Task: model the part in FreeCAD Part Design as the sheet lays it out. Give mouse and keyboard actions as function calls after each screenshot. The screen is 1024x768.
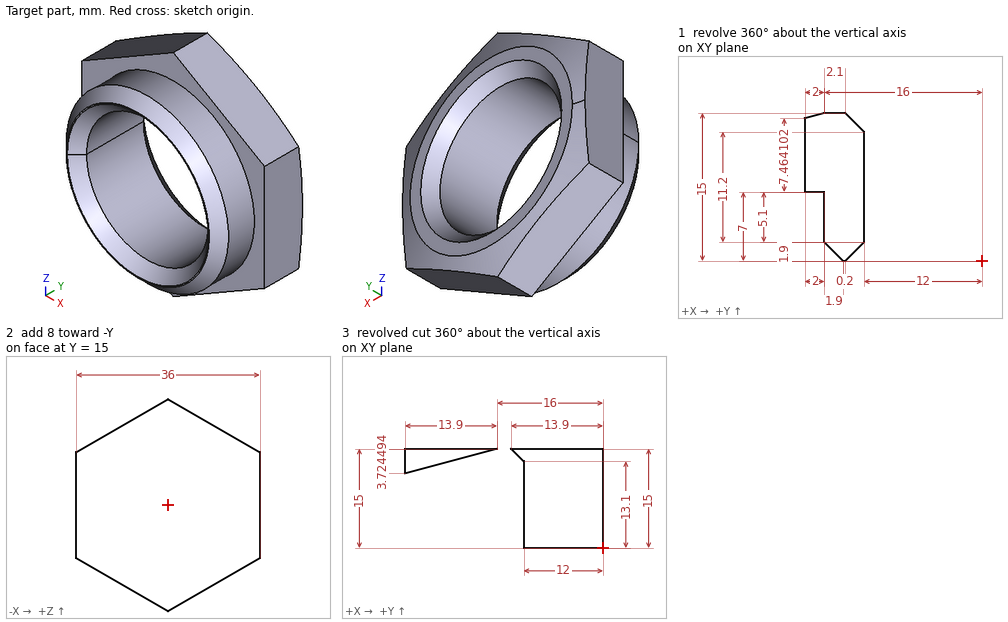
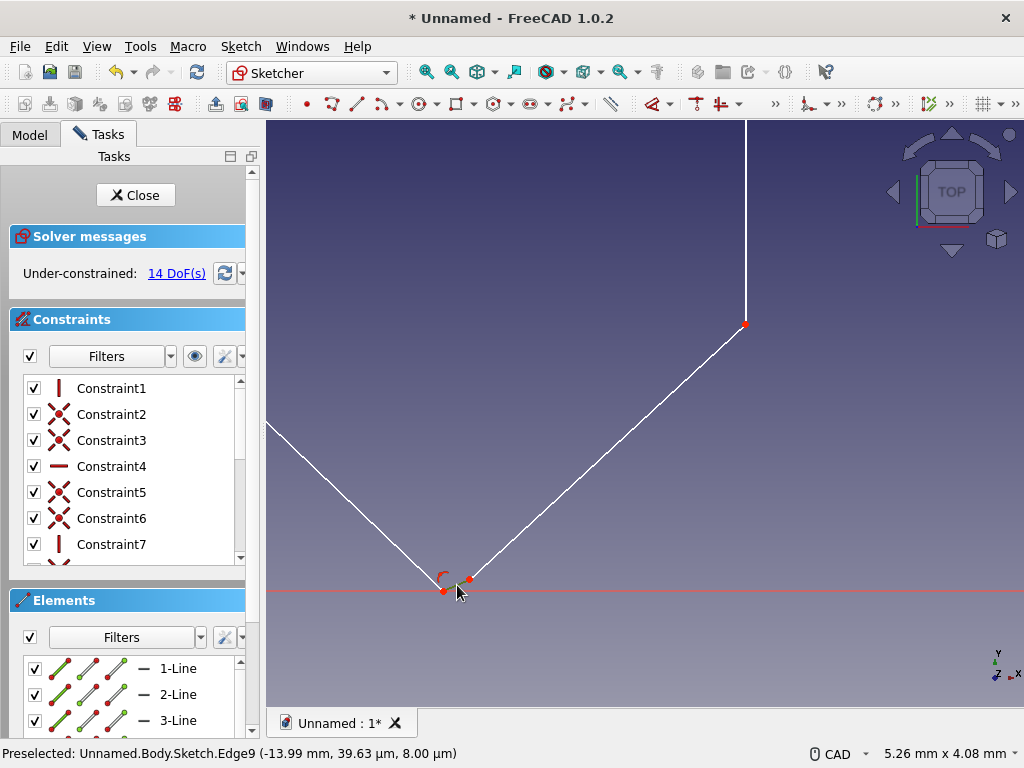
key(h)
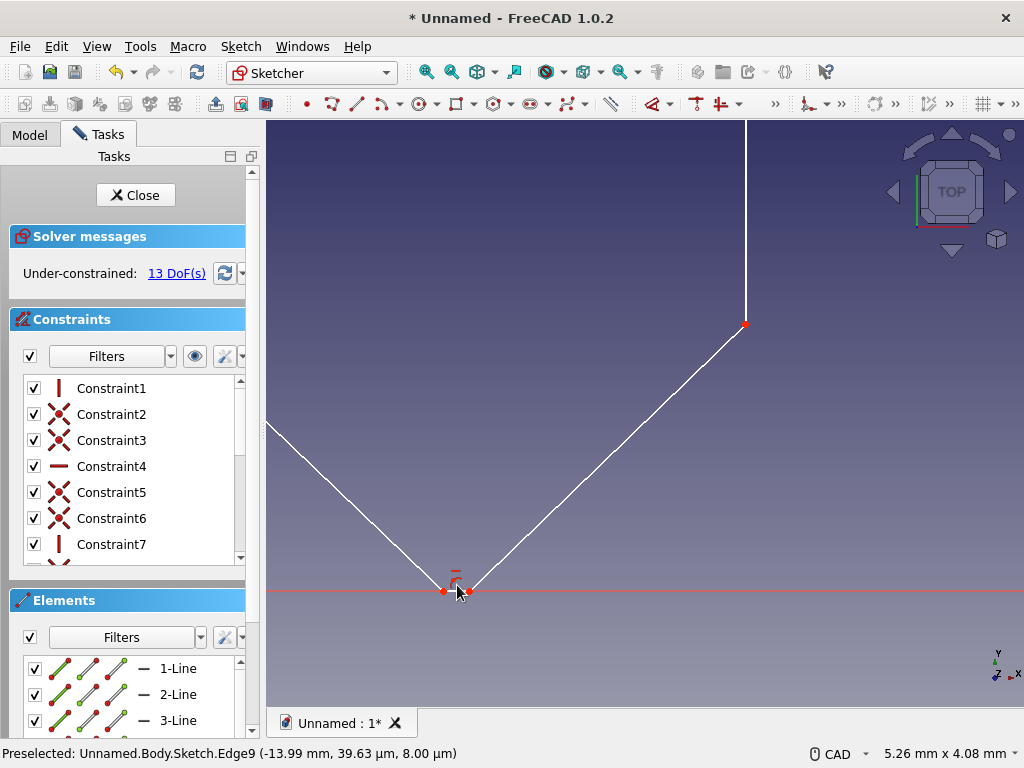
click(652, 104)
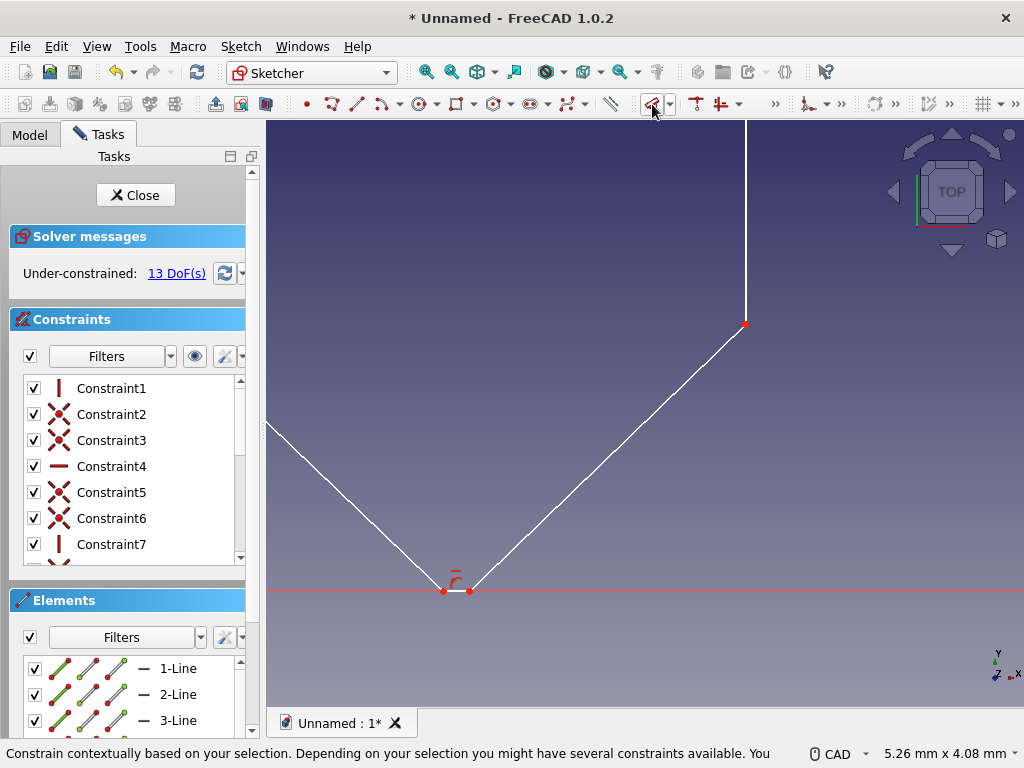
scroll(458, 592, down, 9)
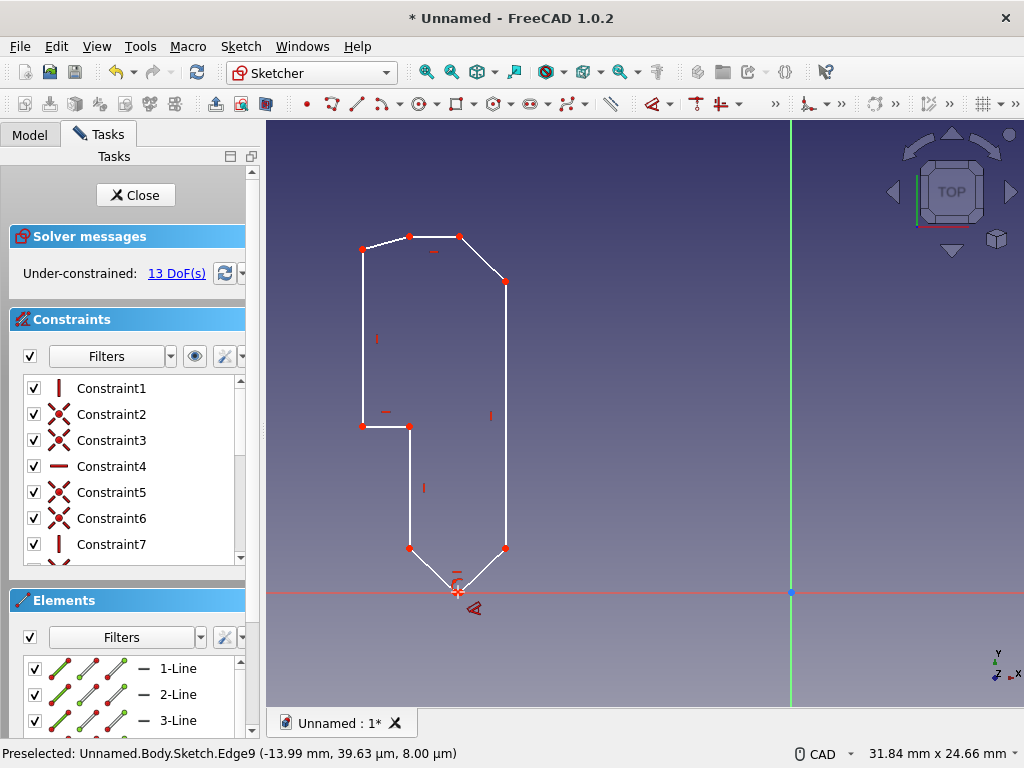
click(377, 427)
click(386, 461)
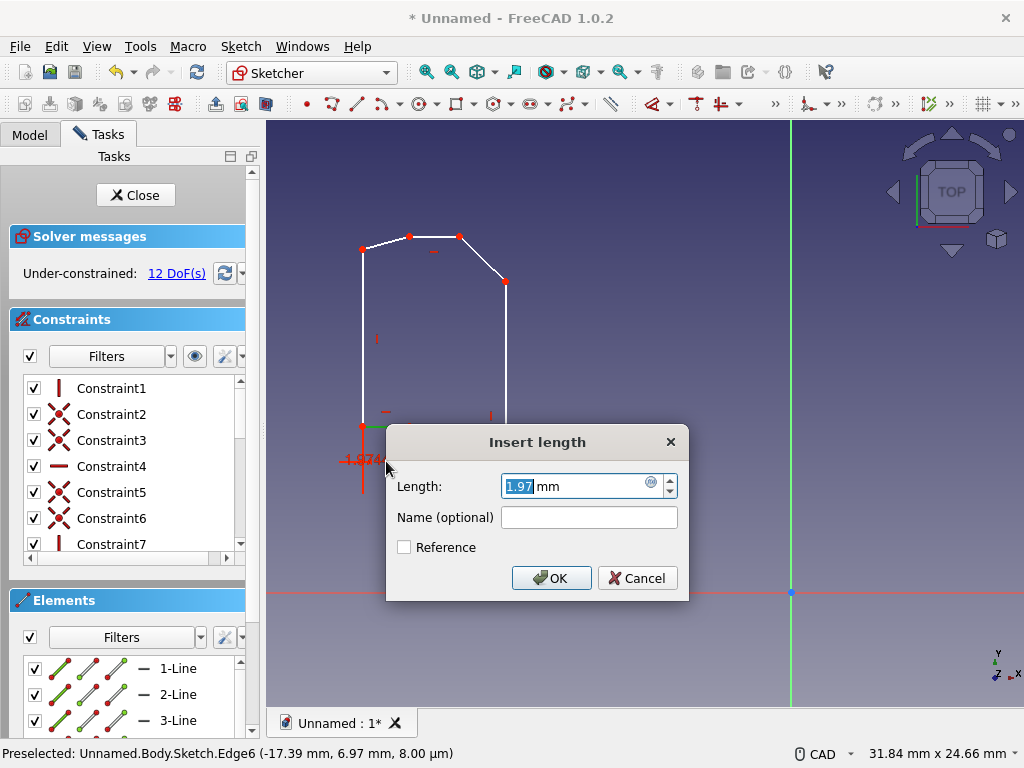
text(2)
key(Return)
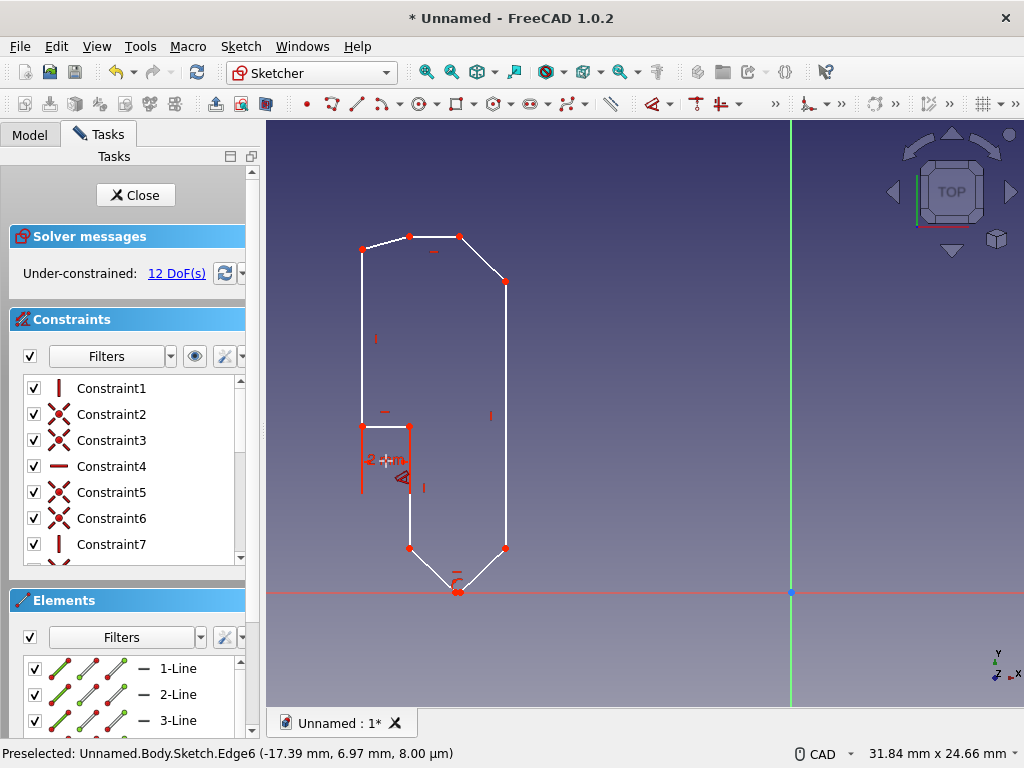
click(362, 427)
click(328, 510)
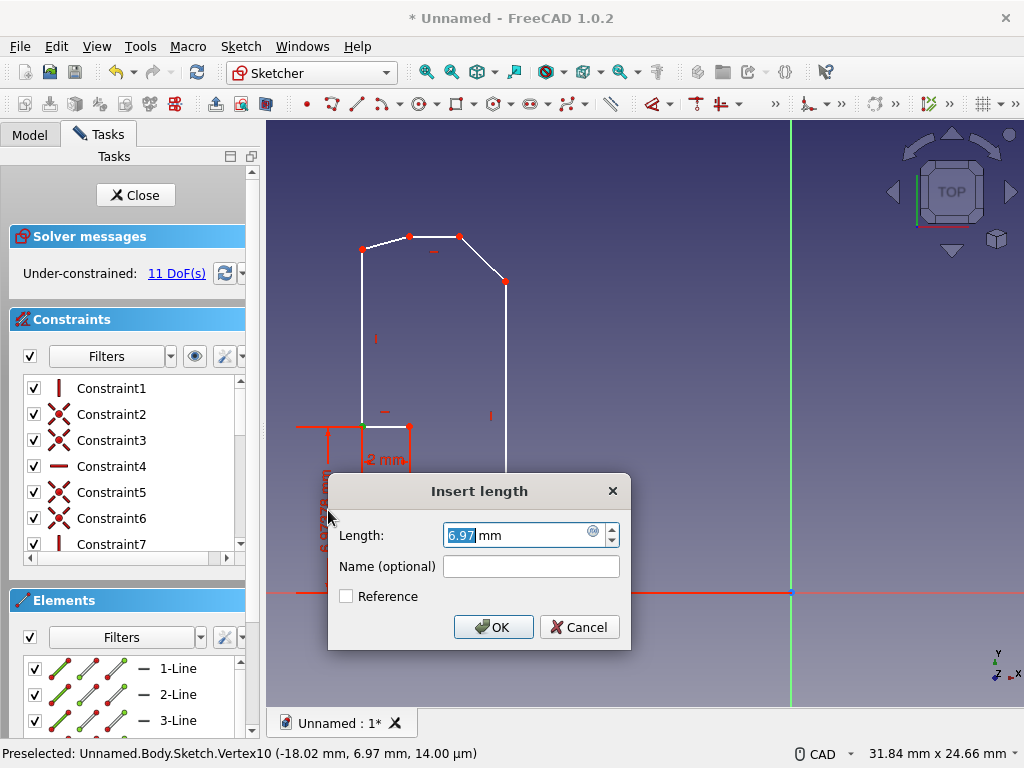
text(7)
key(Return)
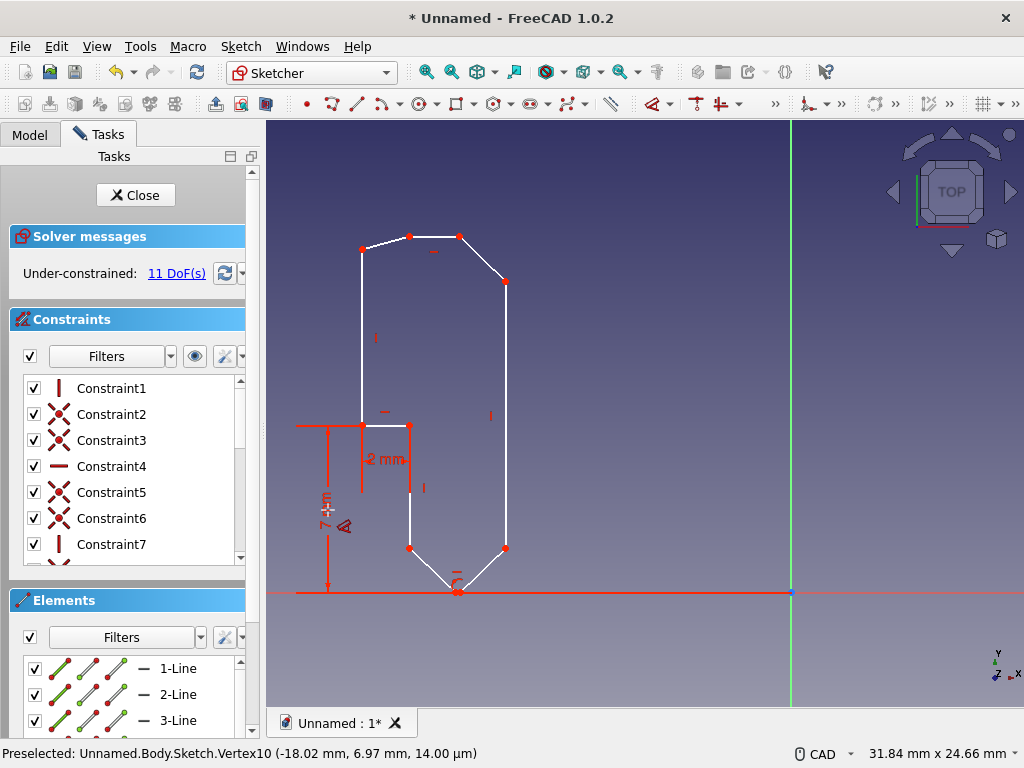
click(395, 240)
click(386, 203)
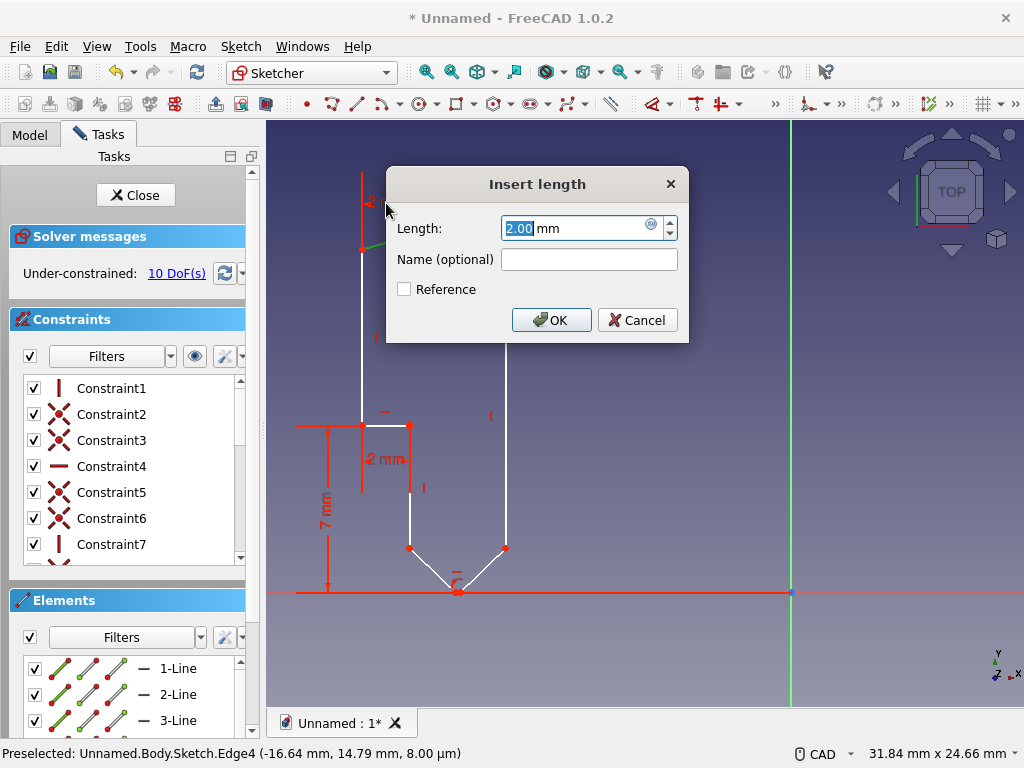
text(2)
key(Return)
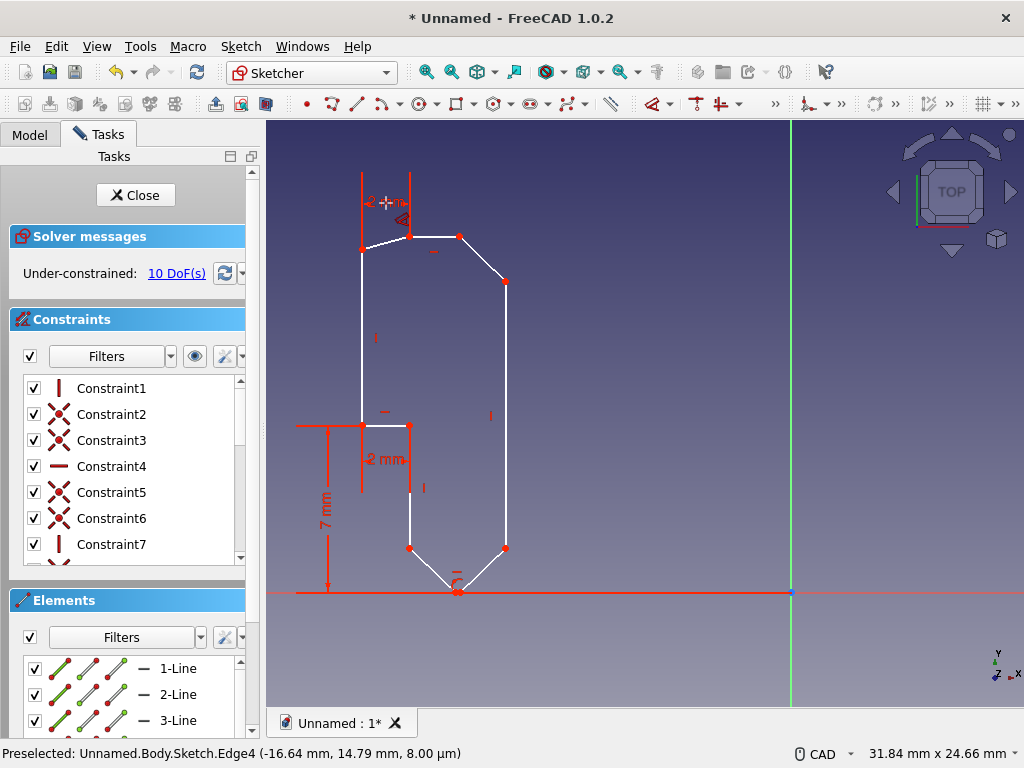
click(445, 237)
click(435, 271)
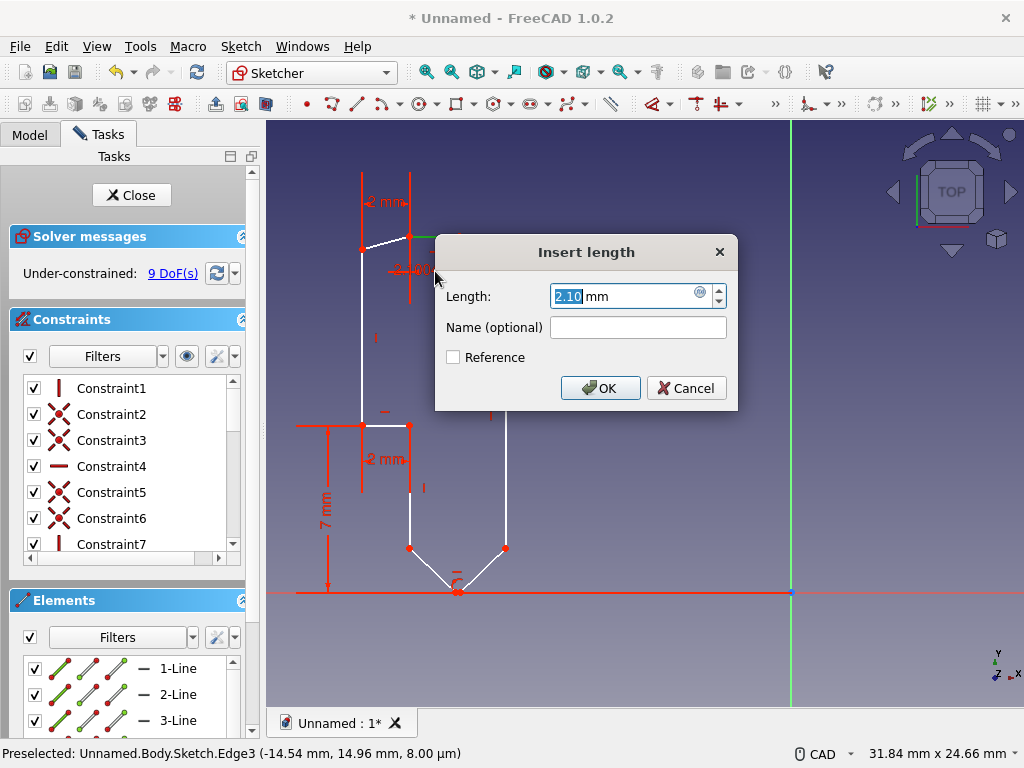
text(2.1)
key(Return)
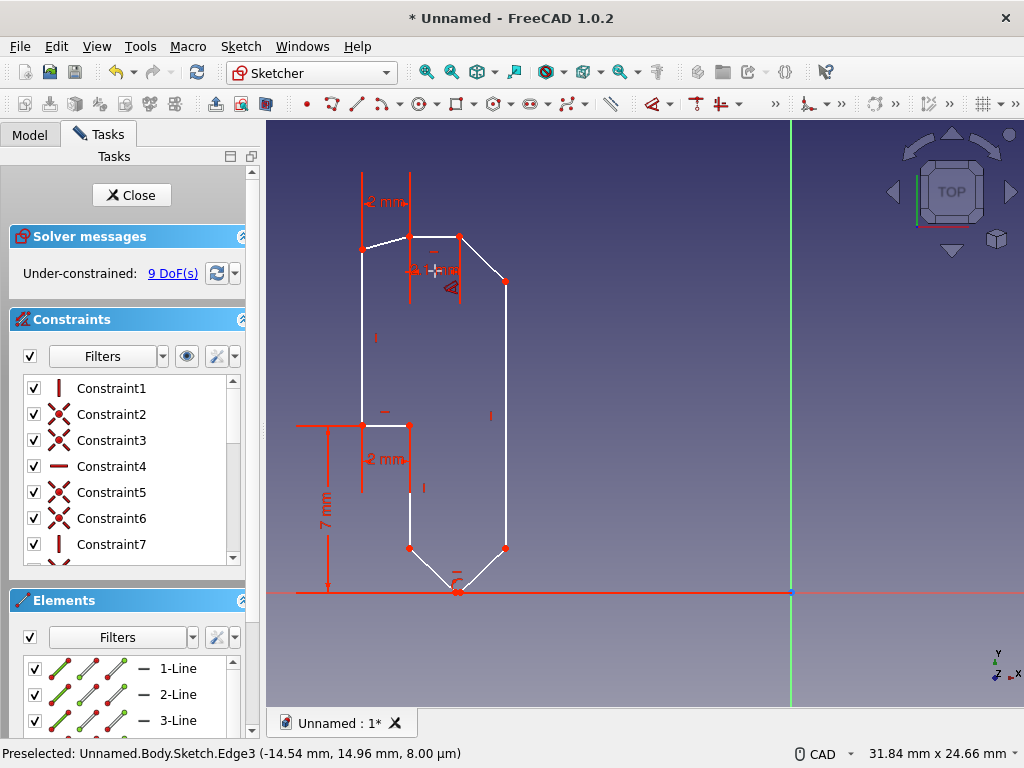
click(410, 463)
click(376, 487)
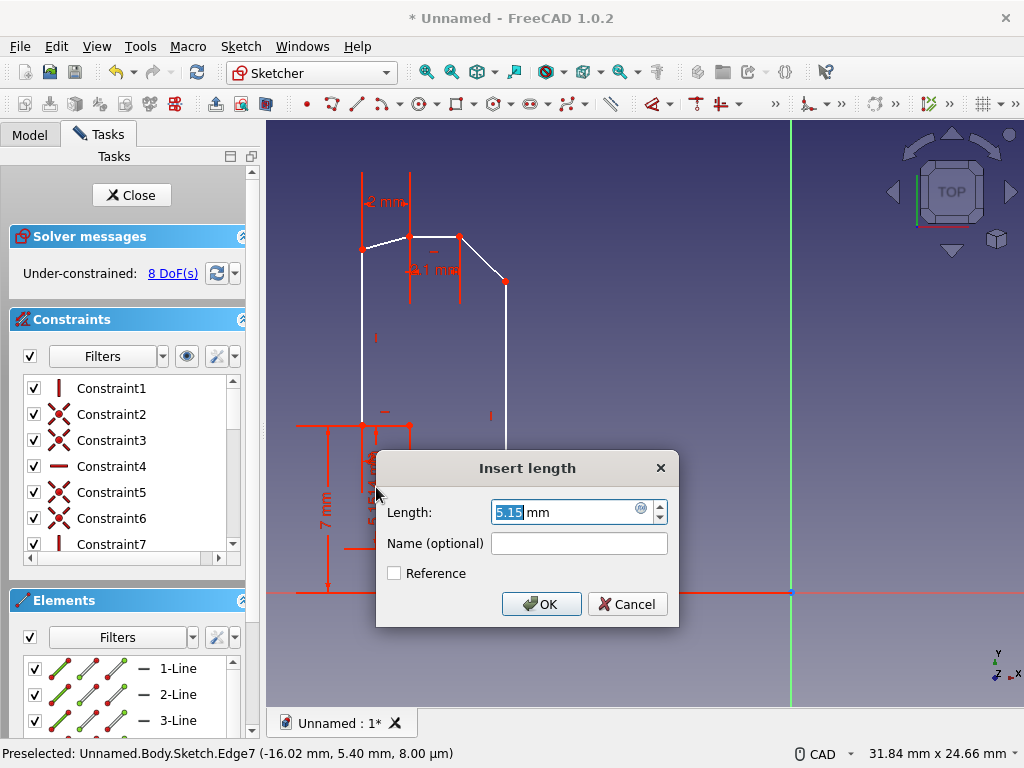
text(5.1)
key(Return)